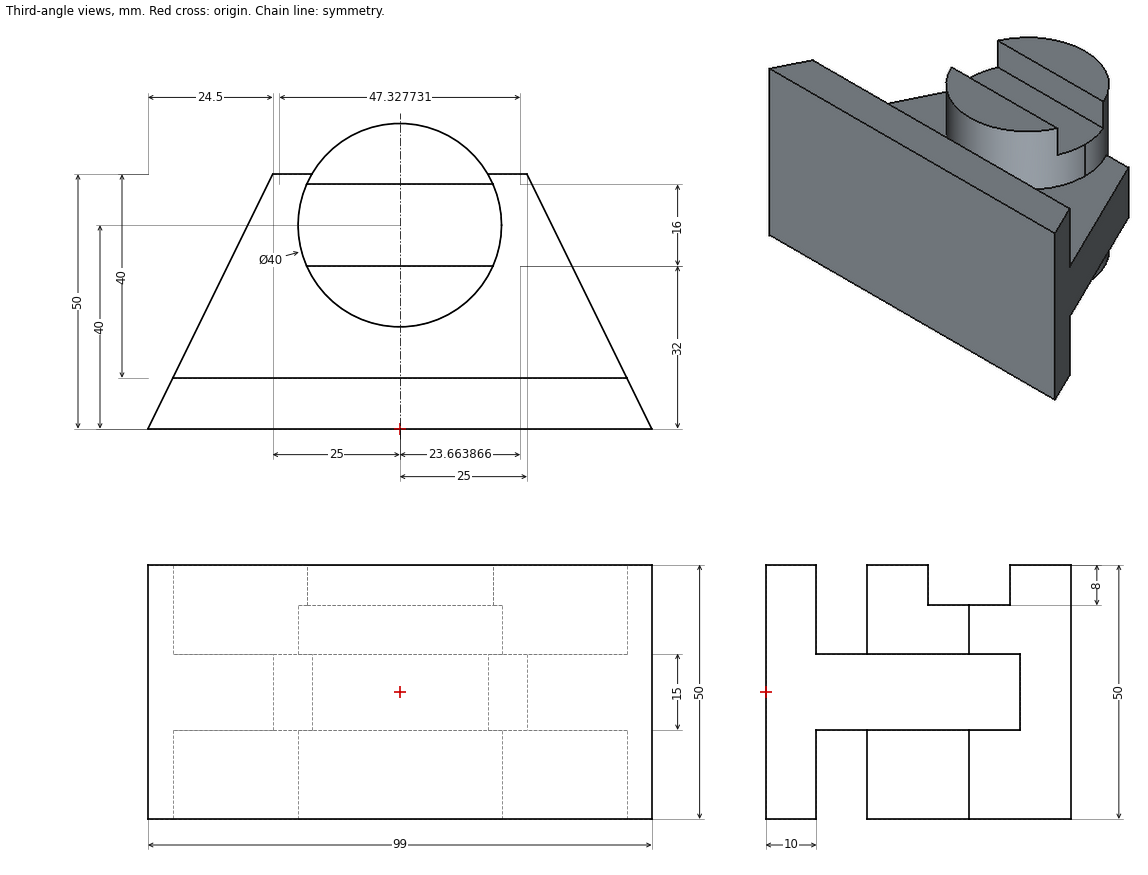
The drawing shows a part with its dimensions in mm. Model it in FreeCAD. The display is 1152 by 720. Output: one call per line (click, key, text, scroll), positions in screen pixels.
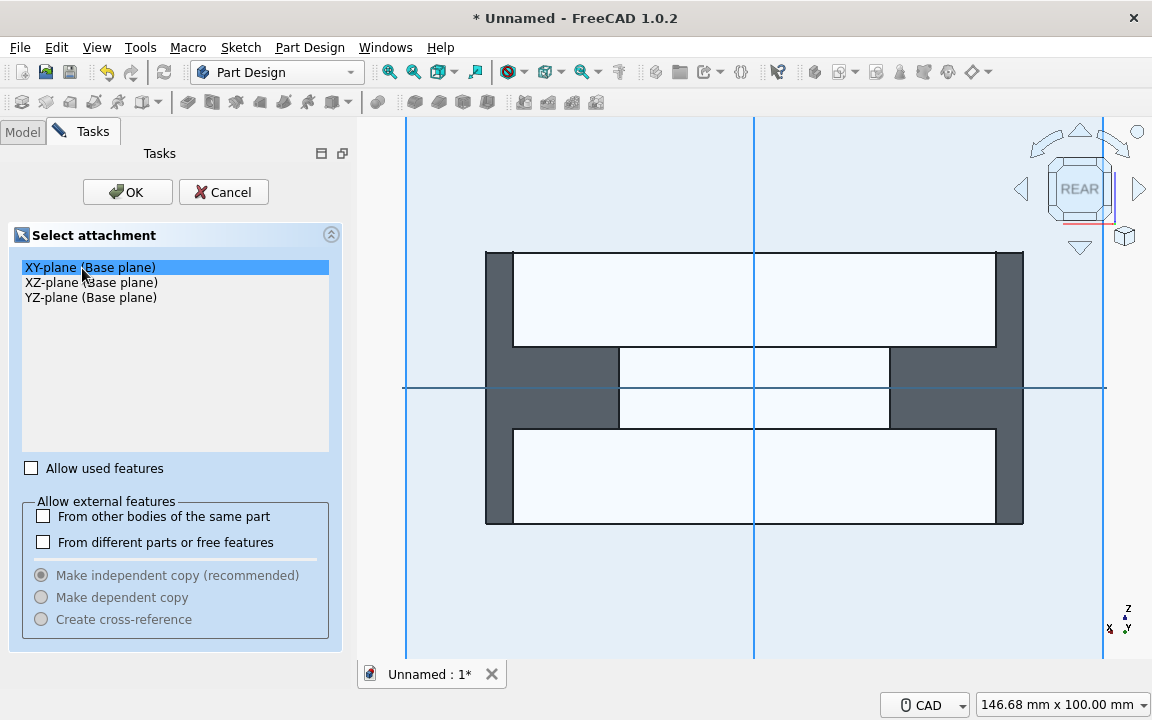
click(128, 192)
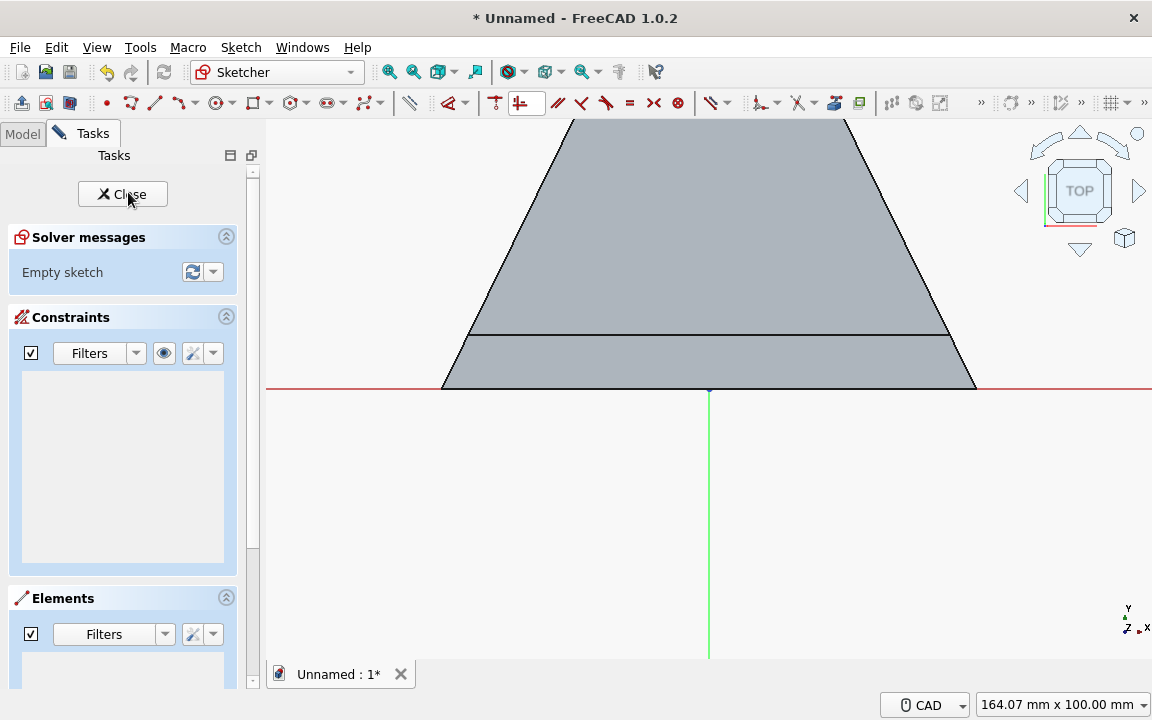
key(q)
key(s)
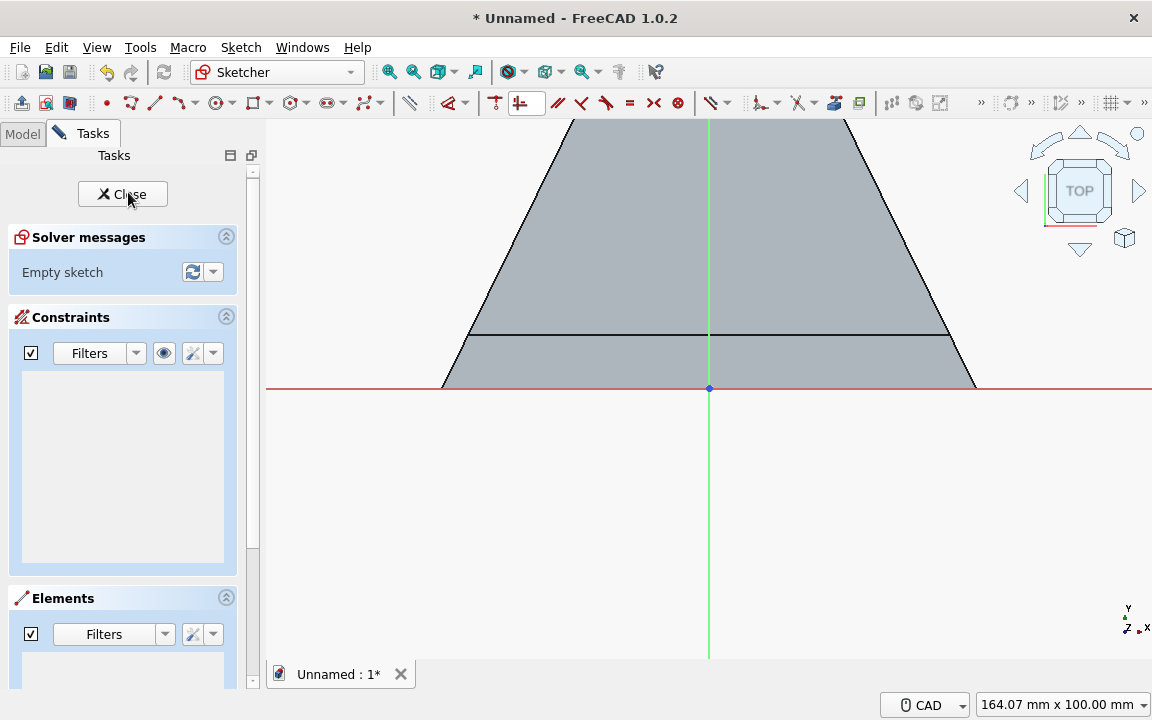
scroll(501, 631, down, 2)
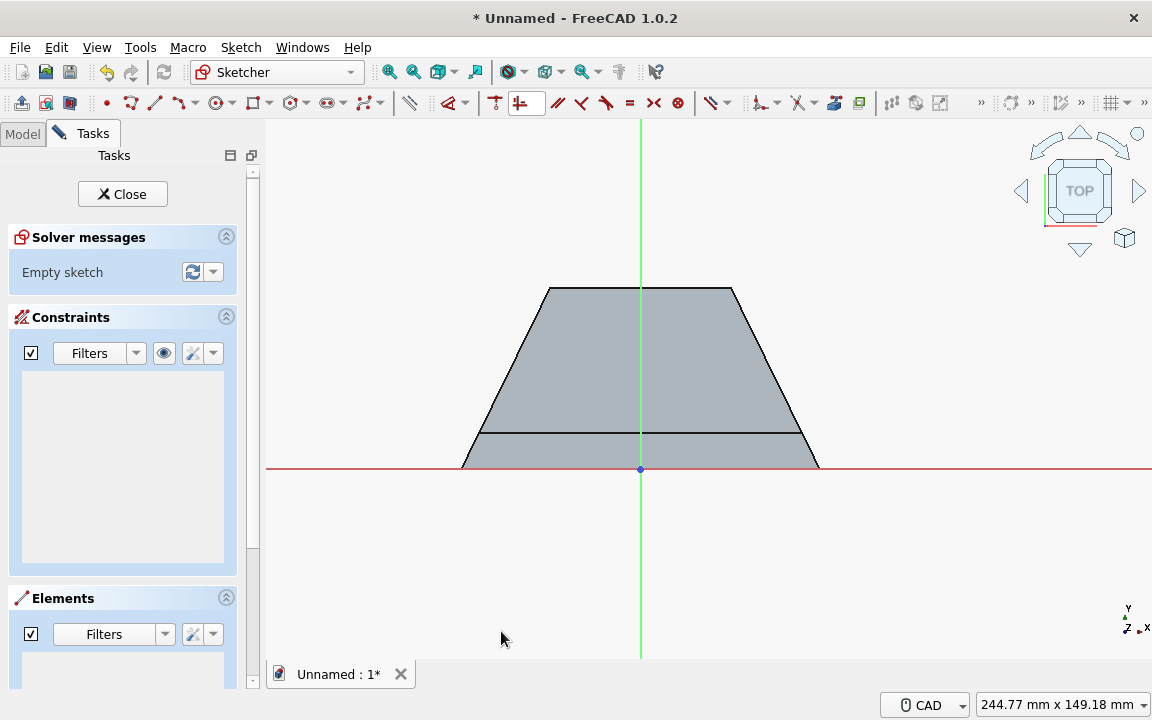
scroll(641, 303, up, 2)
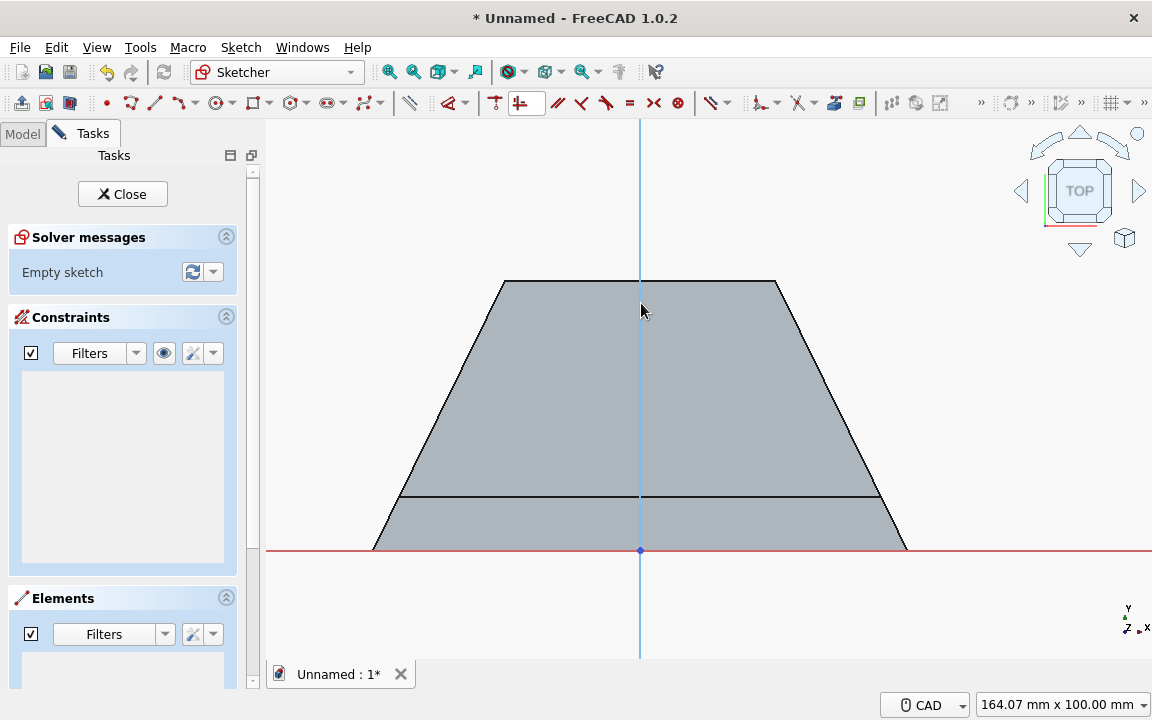
click(216, 104)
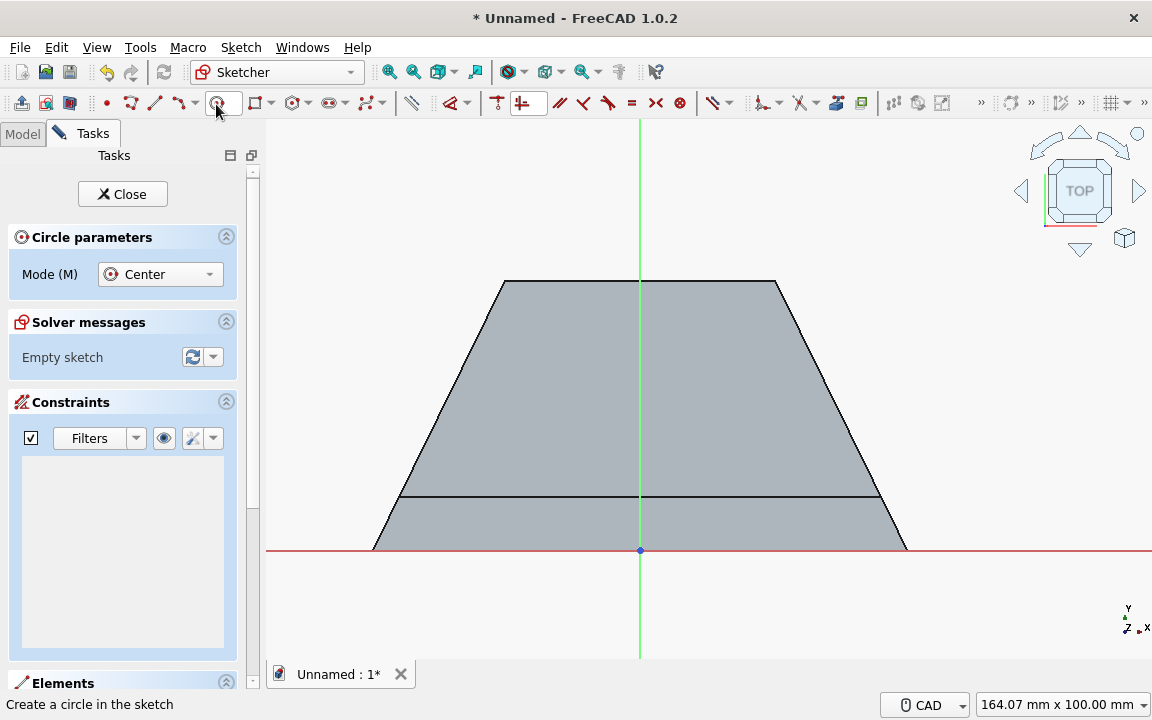
click(640, 335)
click(716, 258)
key(Escape)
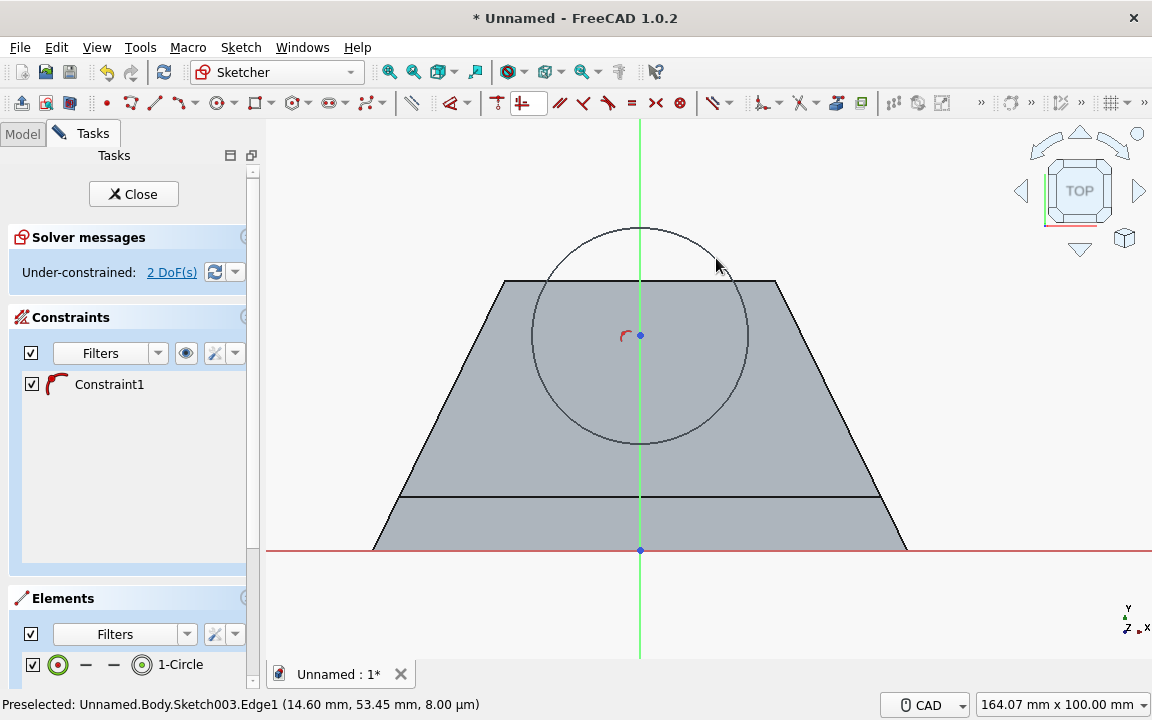
key(d)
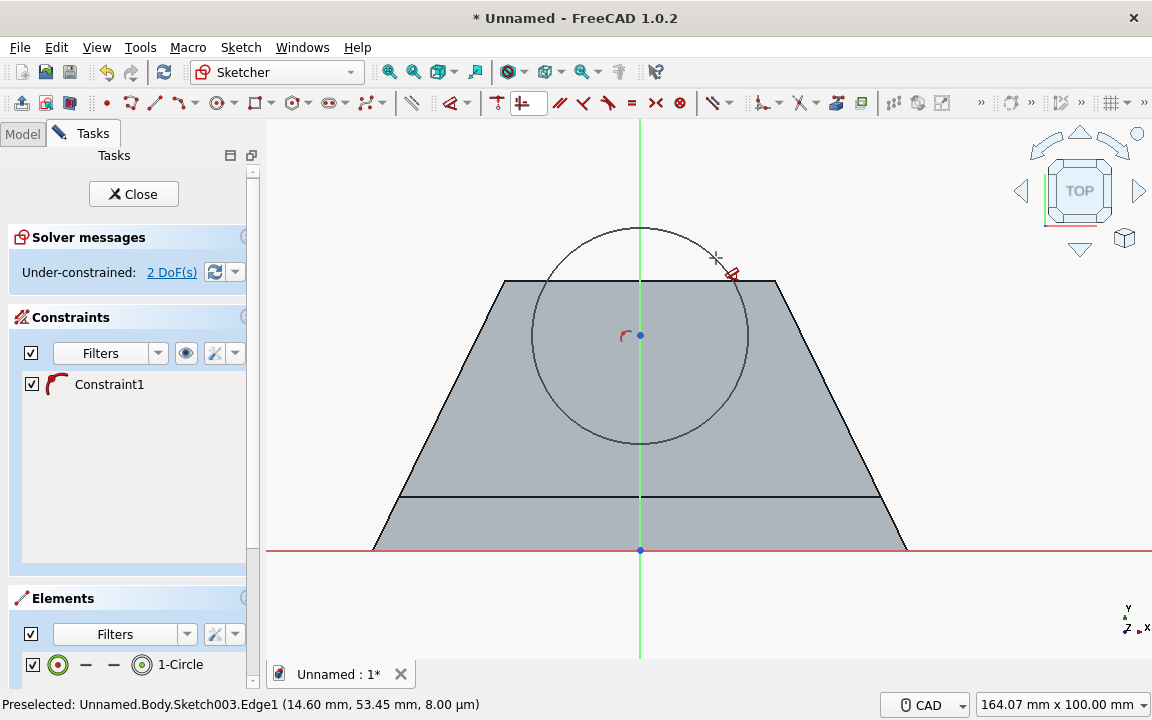
click(716, 259)
click(738, 236)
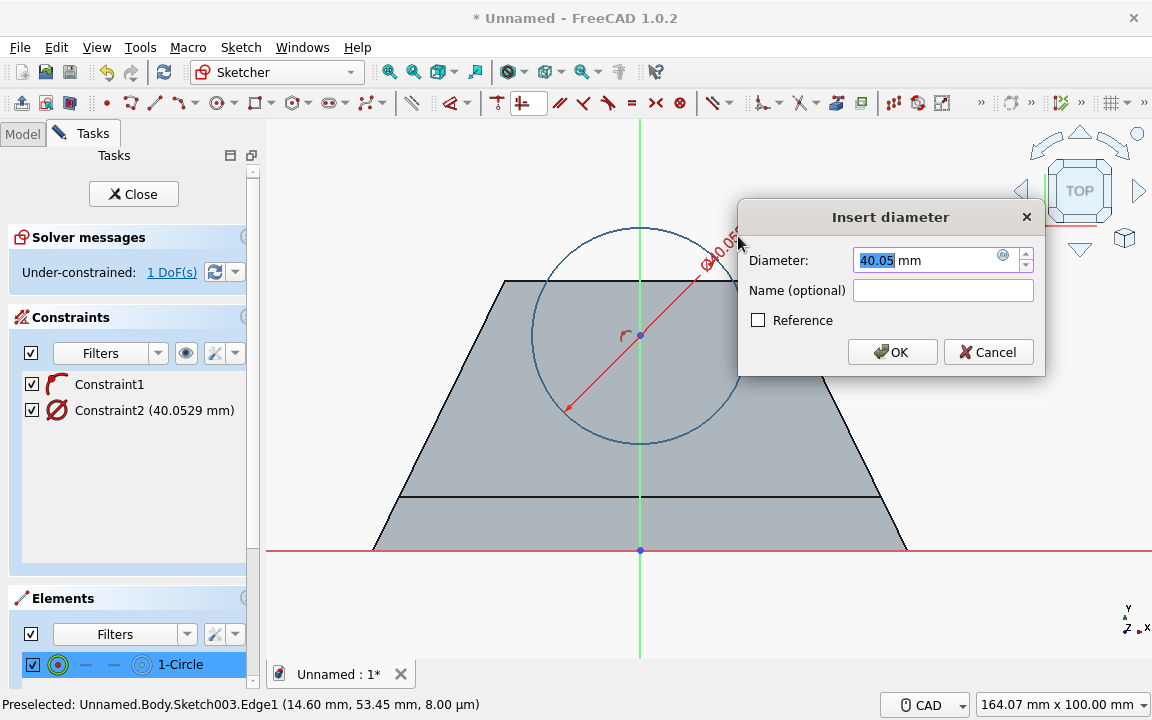
text(40)
key(Return)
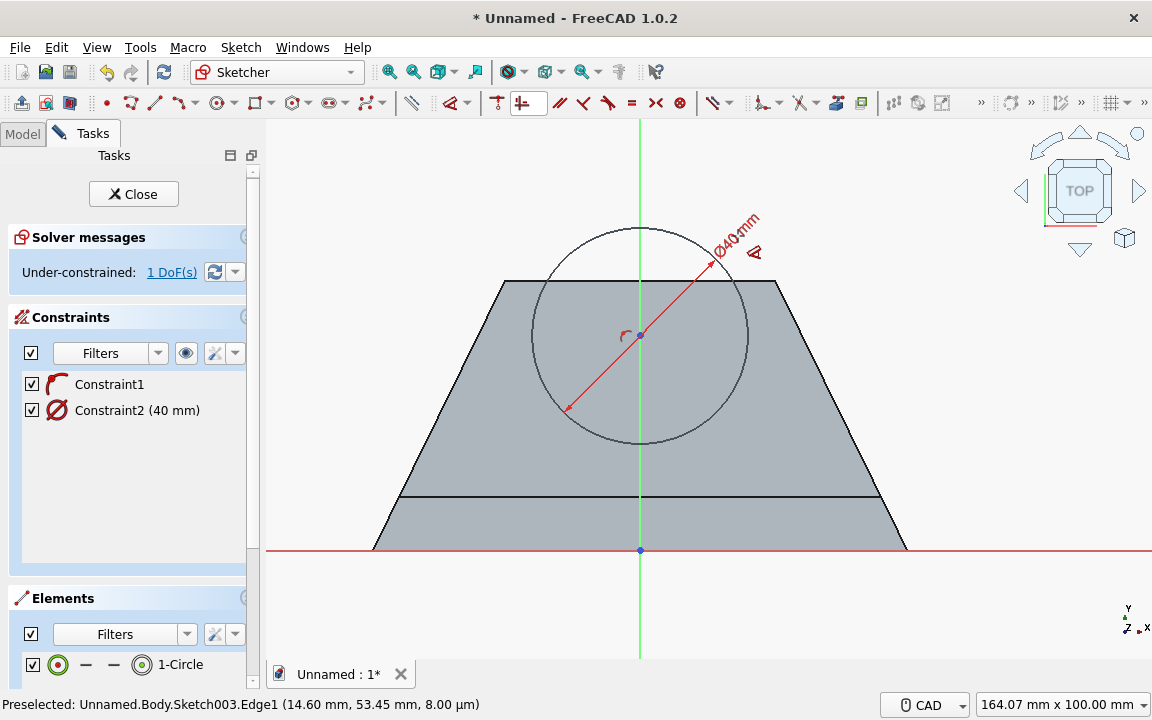
click(640, 336)
click(674, 394)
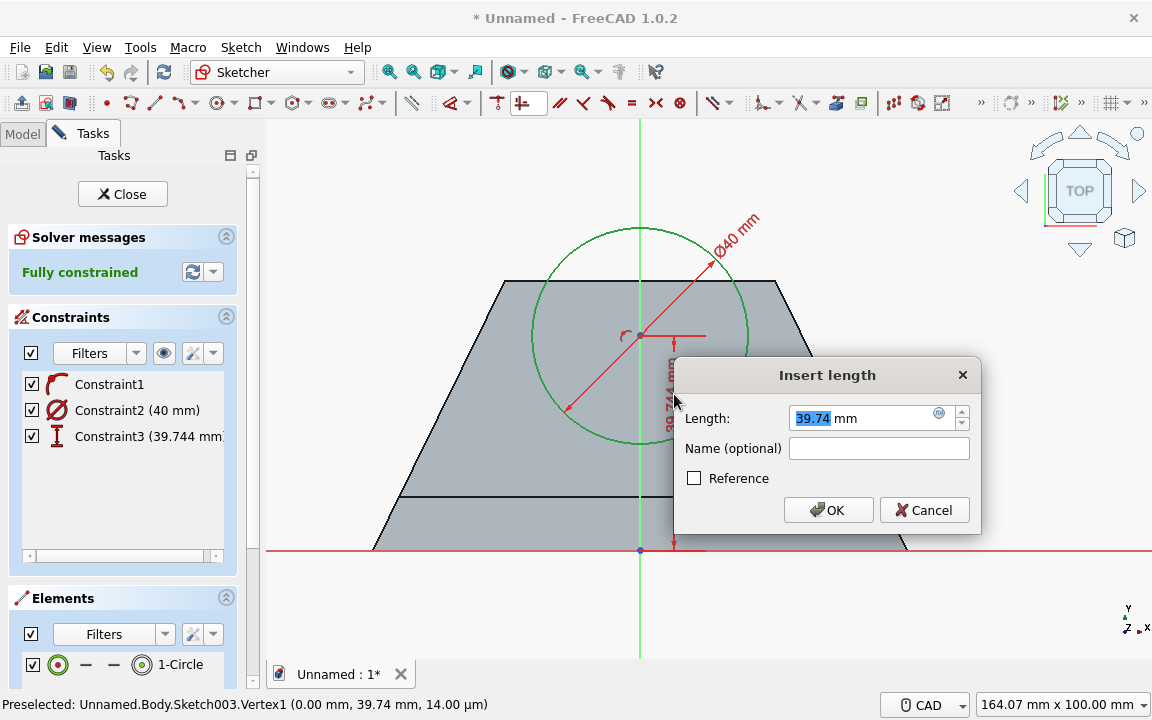
text(40)
key(Return)
key(Escape)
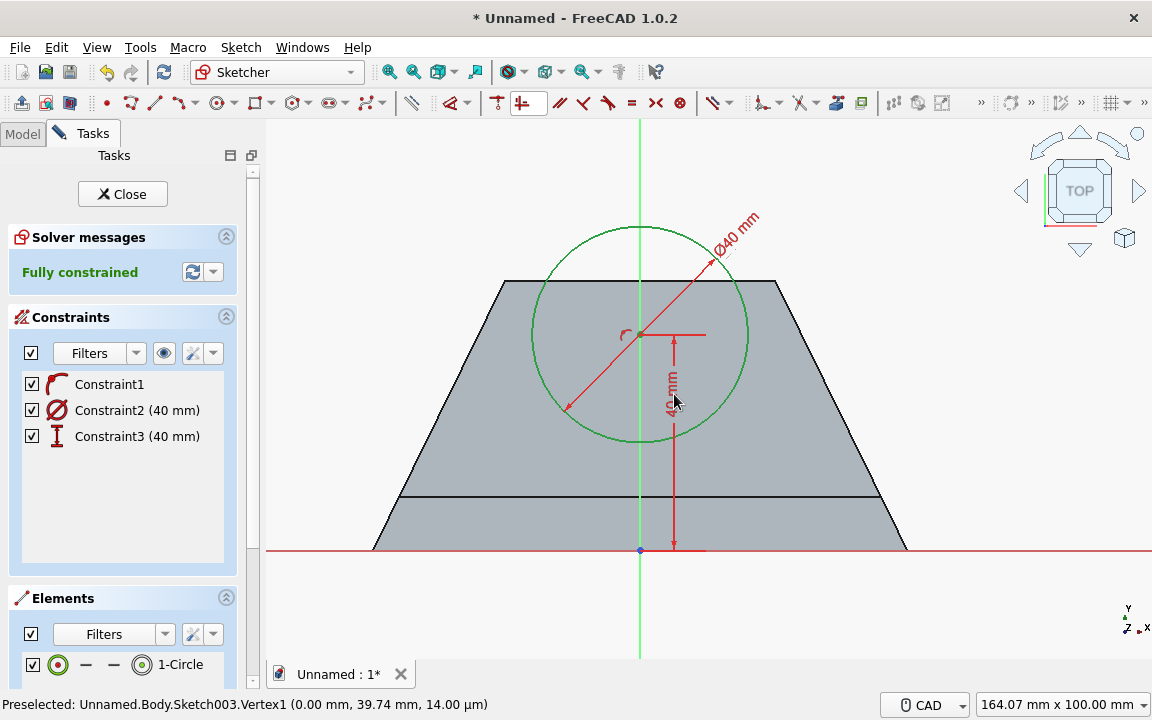
click(123, 194)